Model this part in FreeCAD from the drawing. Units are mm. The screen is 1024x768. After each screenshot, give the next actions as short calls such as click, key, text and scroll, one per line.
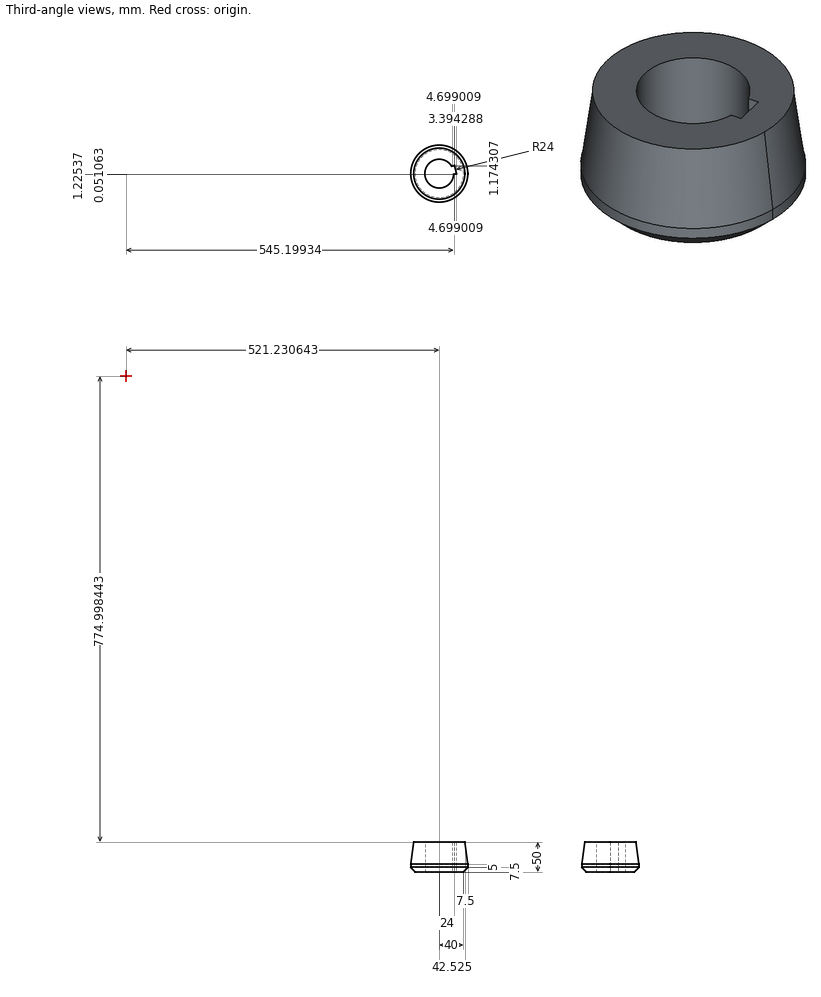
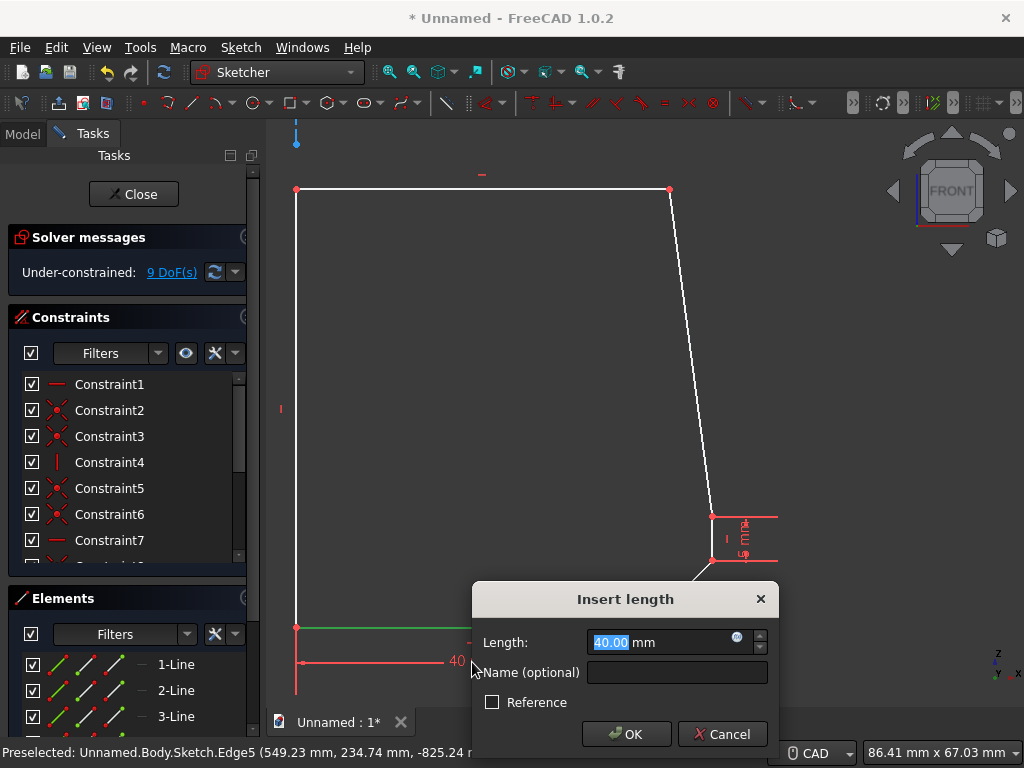
text(40)
key(Return)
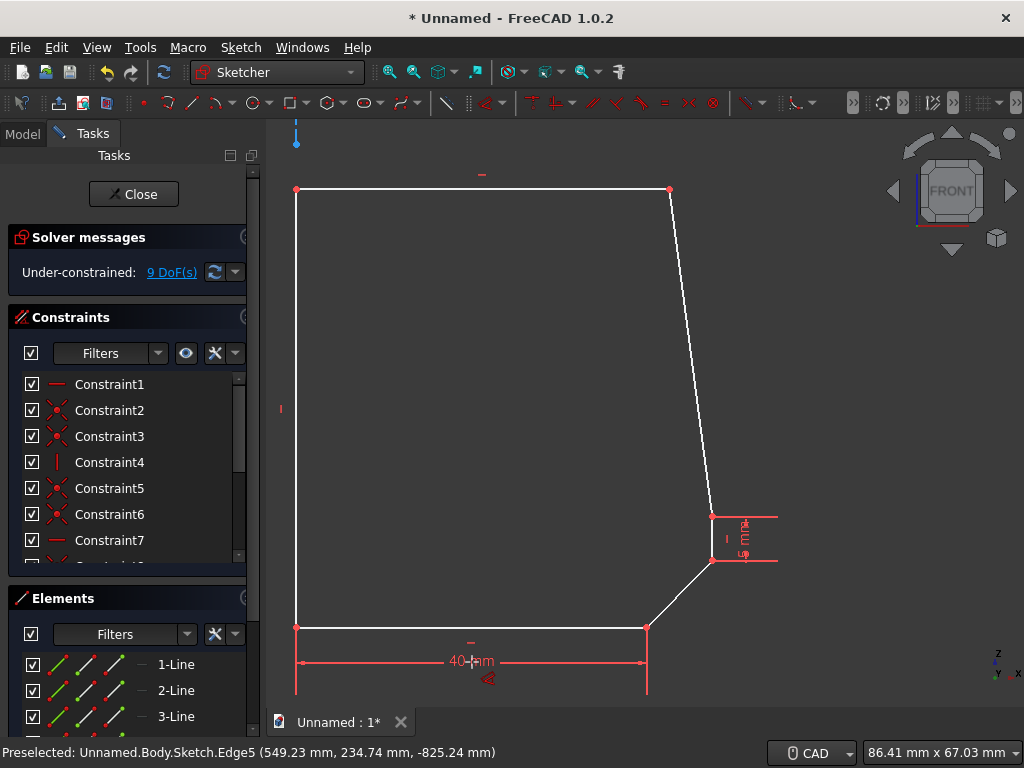
click(296, 496)
click(330, 408)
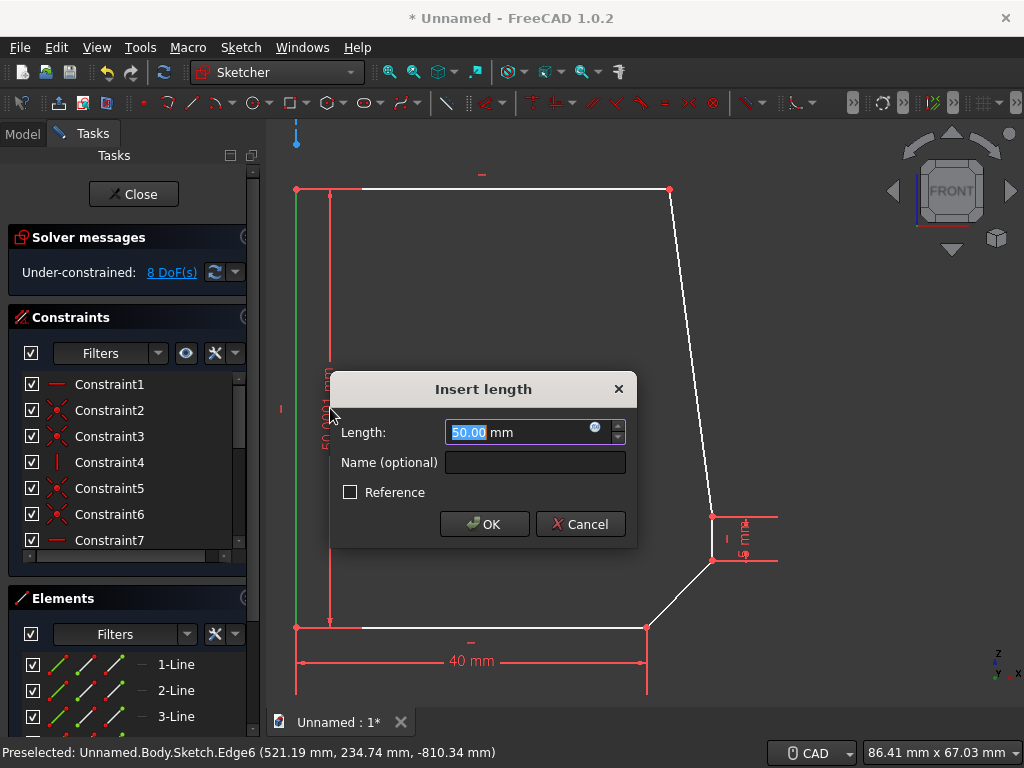
text(50)
key(Return)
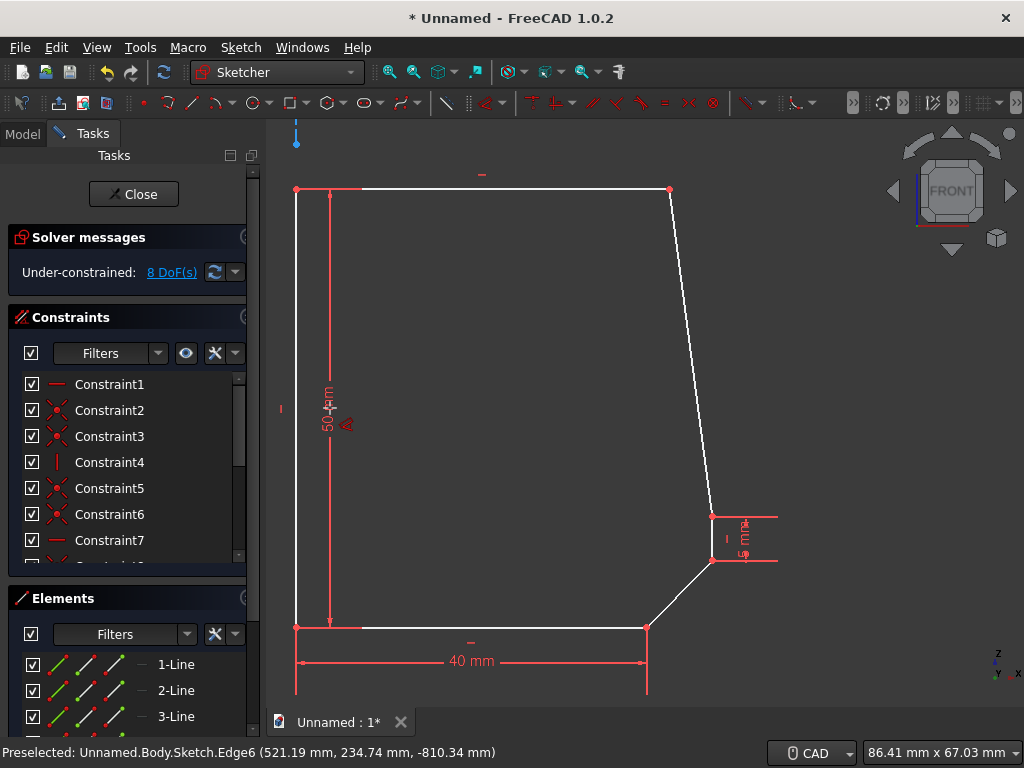
click(693, 581)
click(680, 662)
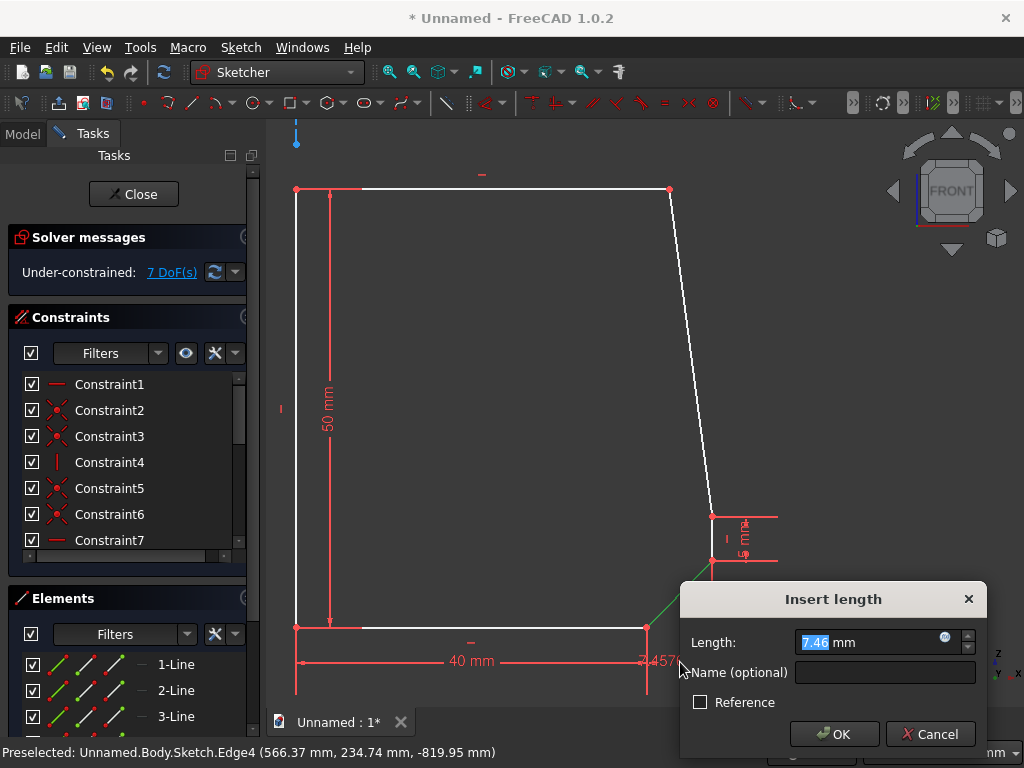
text(7.5)
key(Return)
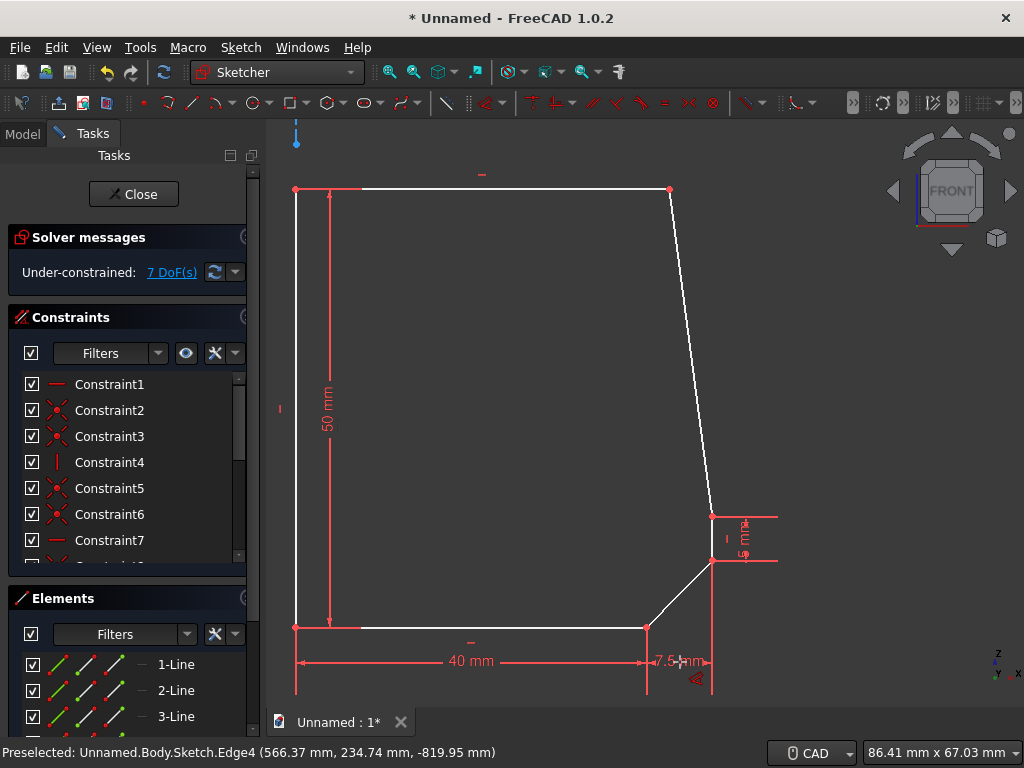
click(693, 581)
click(746, 594)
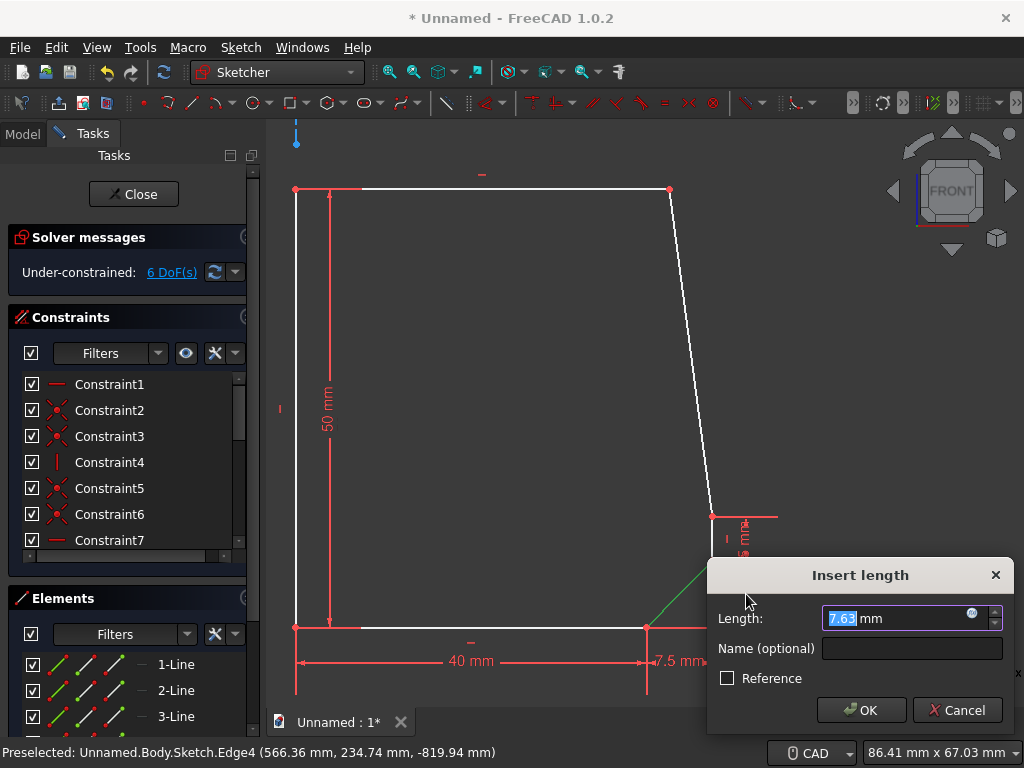
text(7.5)
key(Return)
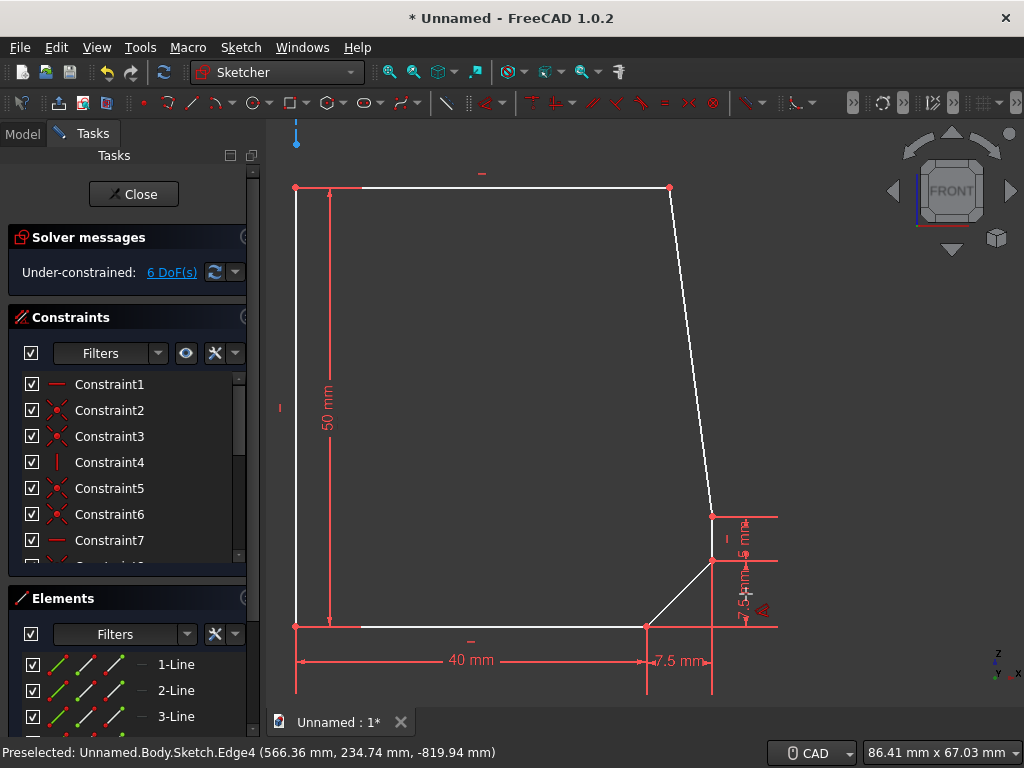
click(408, 188)
click(482, 154)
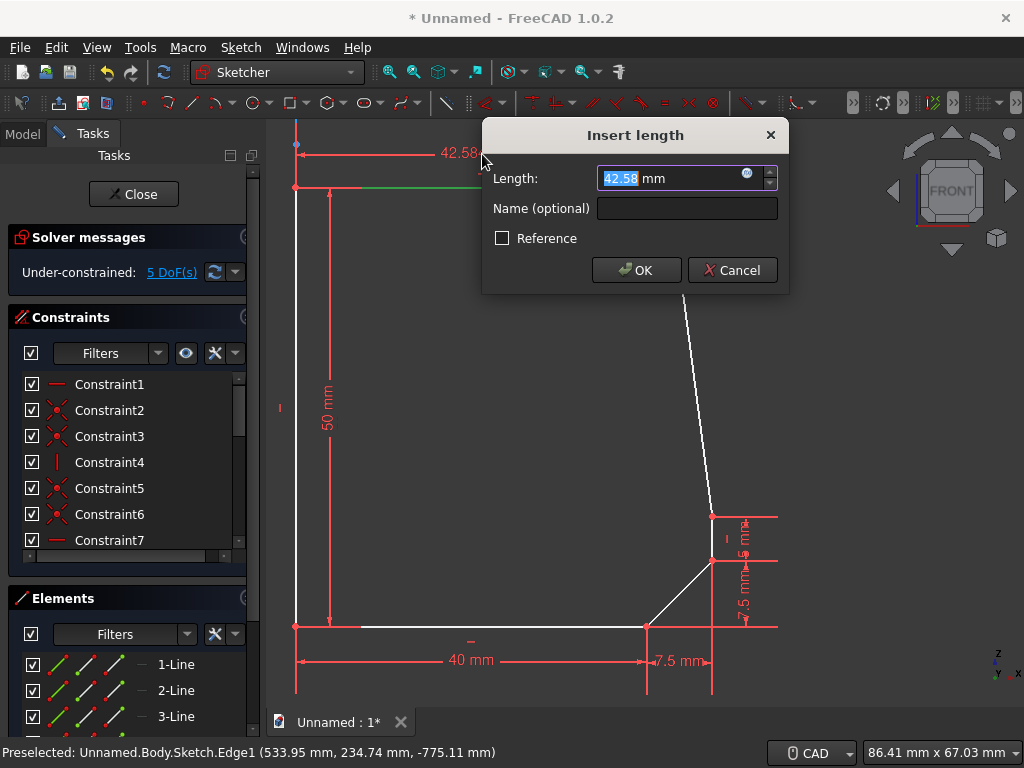
text(42.525)
key(Return)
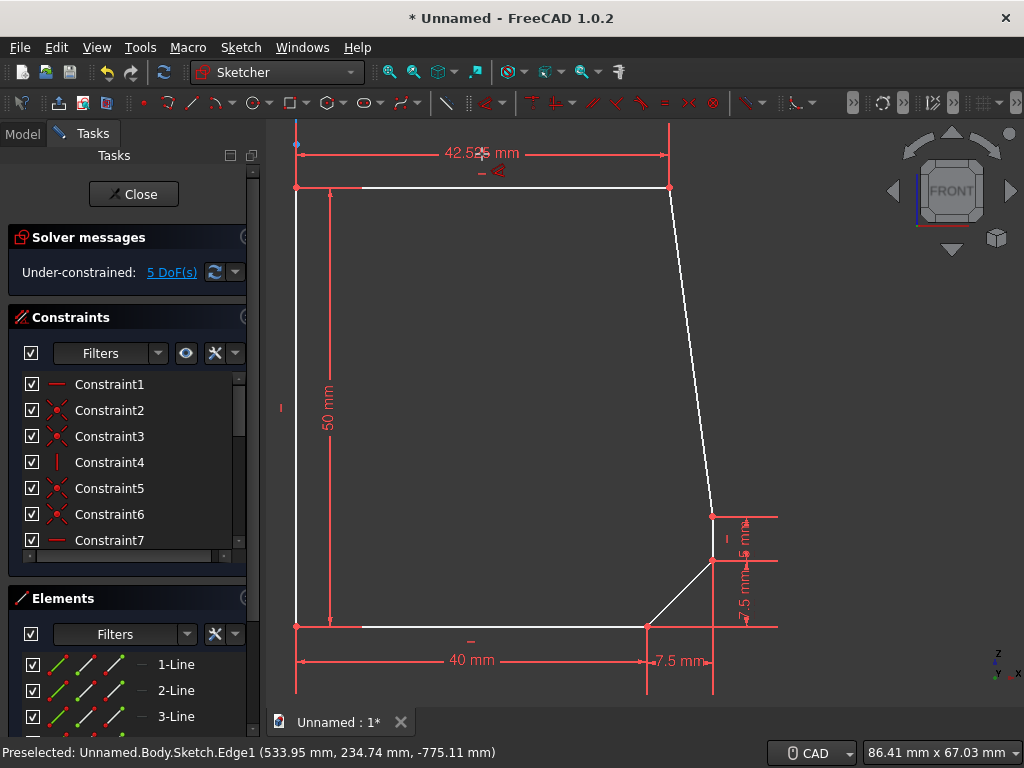
click(296, 188)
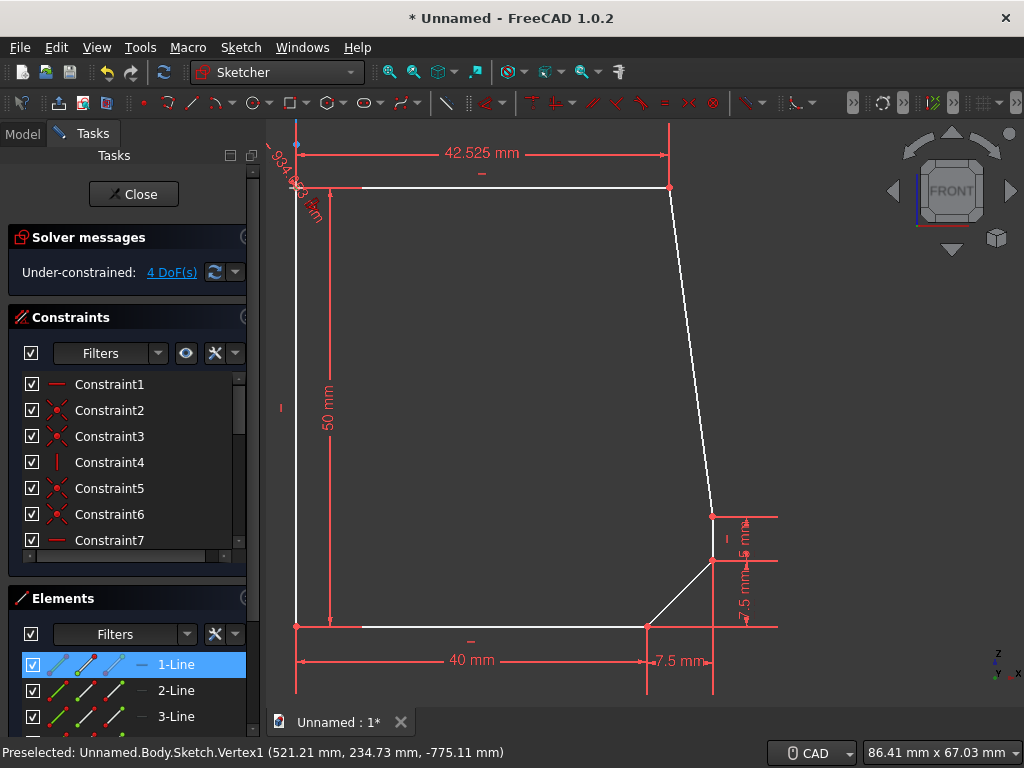
key(Escape)
key(Escape)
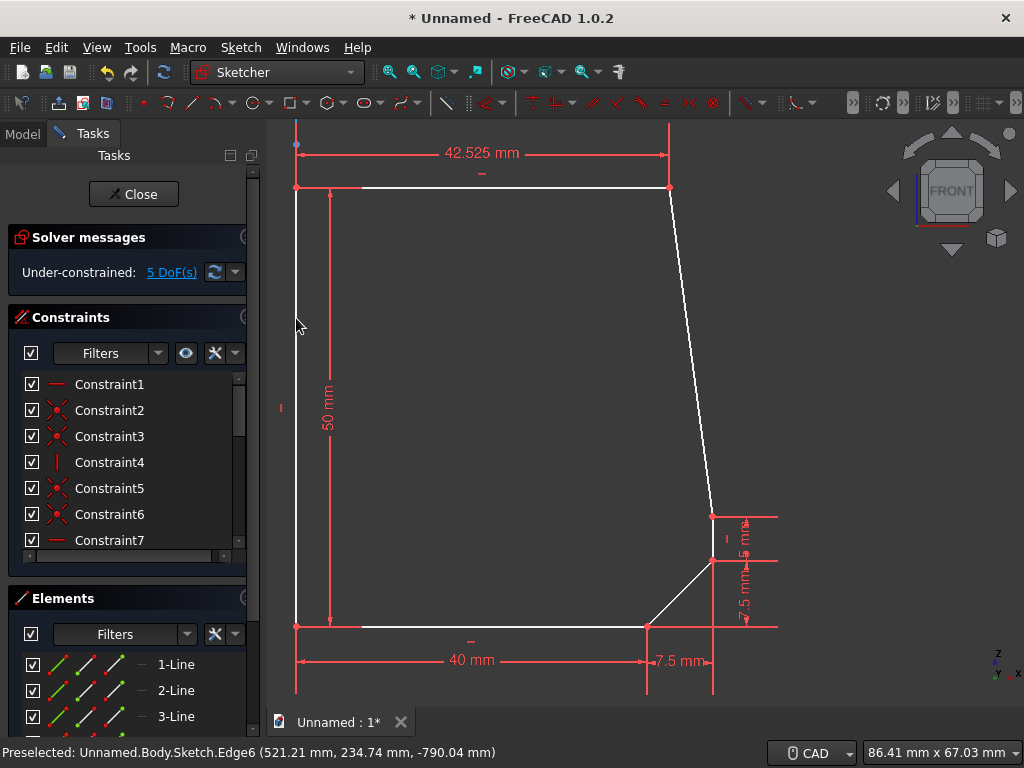
click(296, 188)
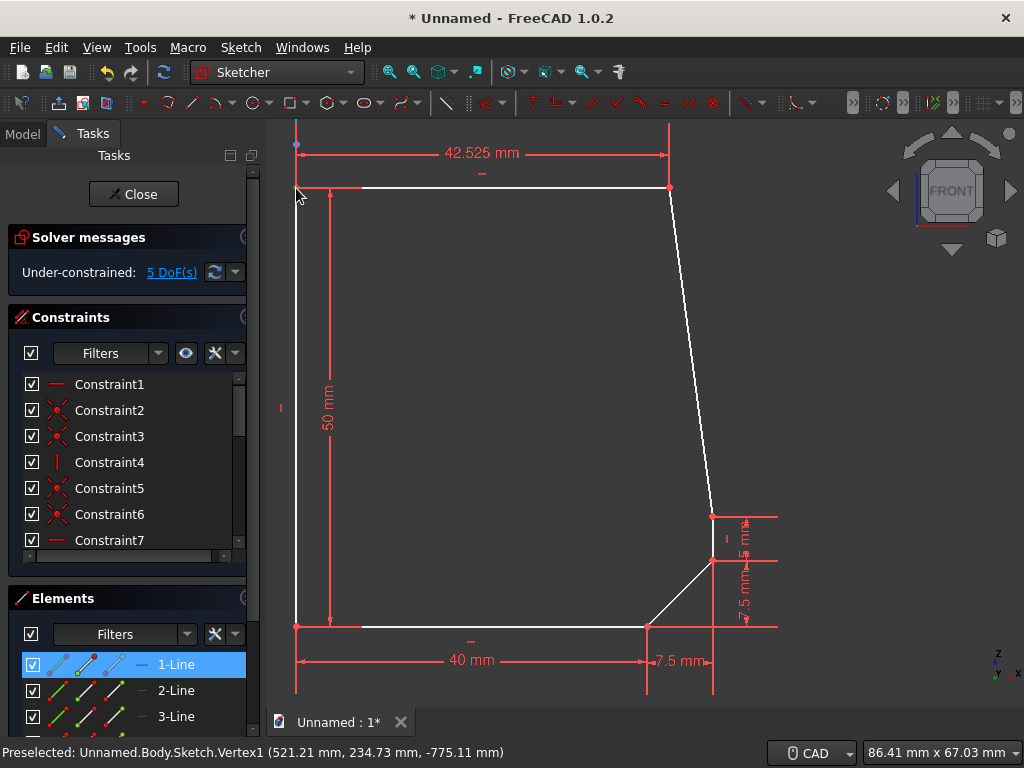
click(504, 104)